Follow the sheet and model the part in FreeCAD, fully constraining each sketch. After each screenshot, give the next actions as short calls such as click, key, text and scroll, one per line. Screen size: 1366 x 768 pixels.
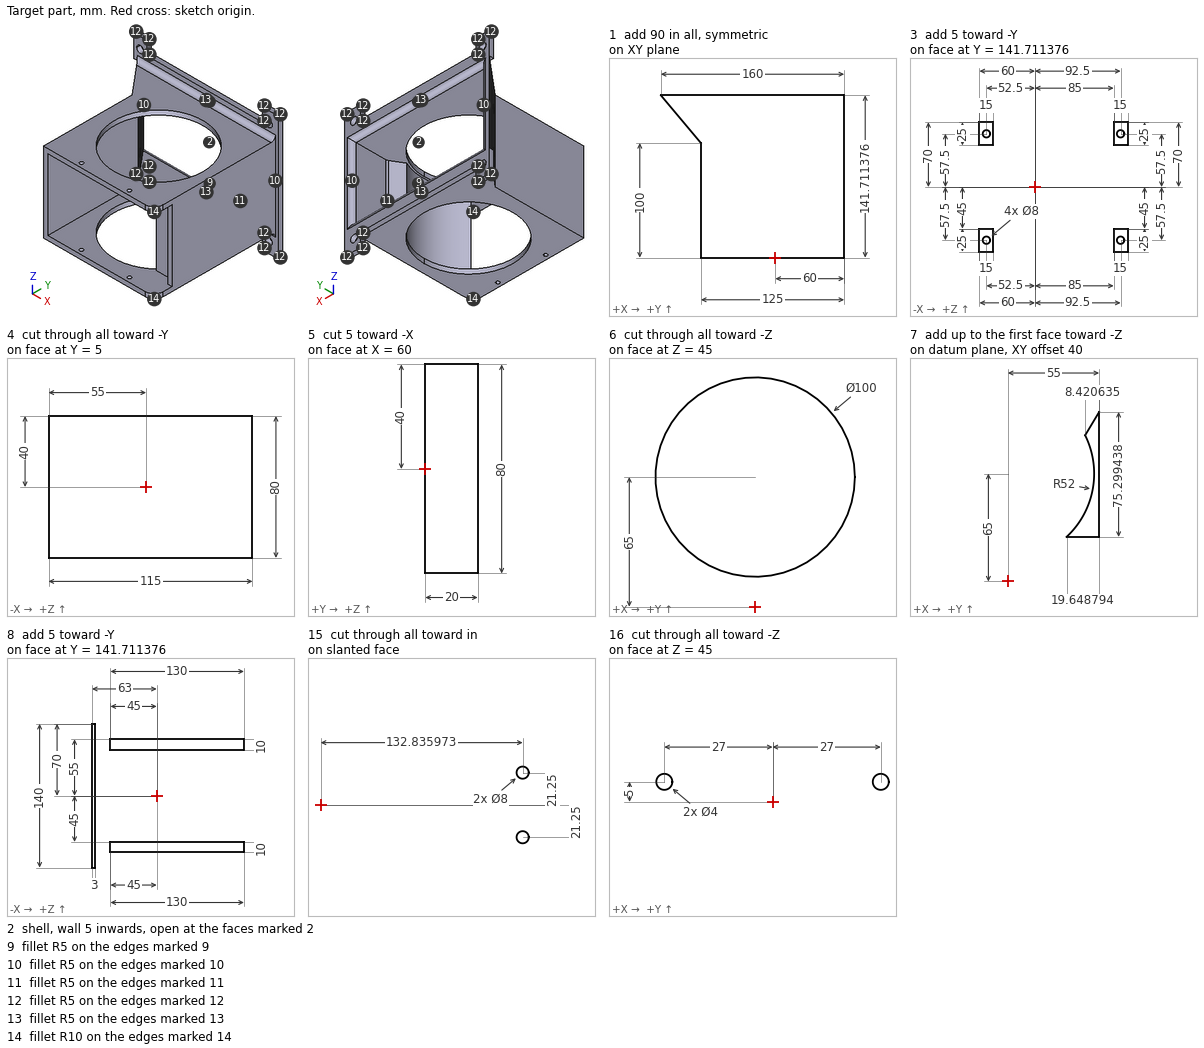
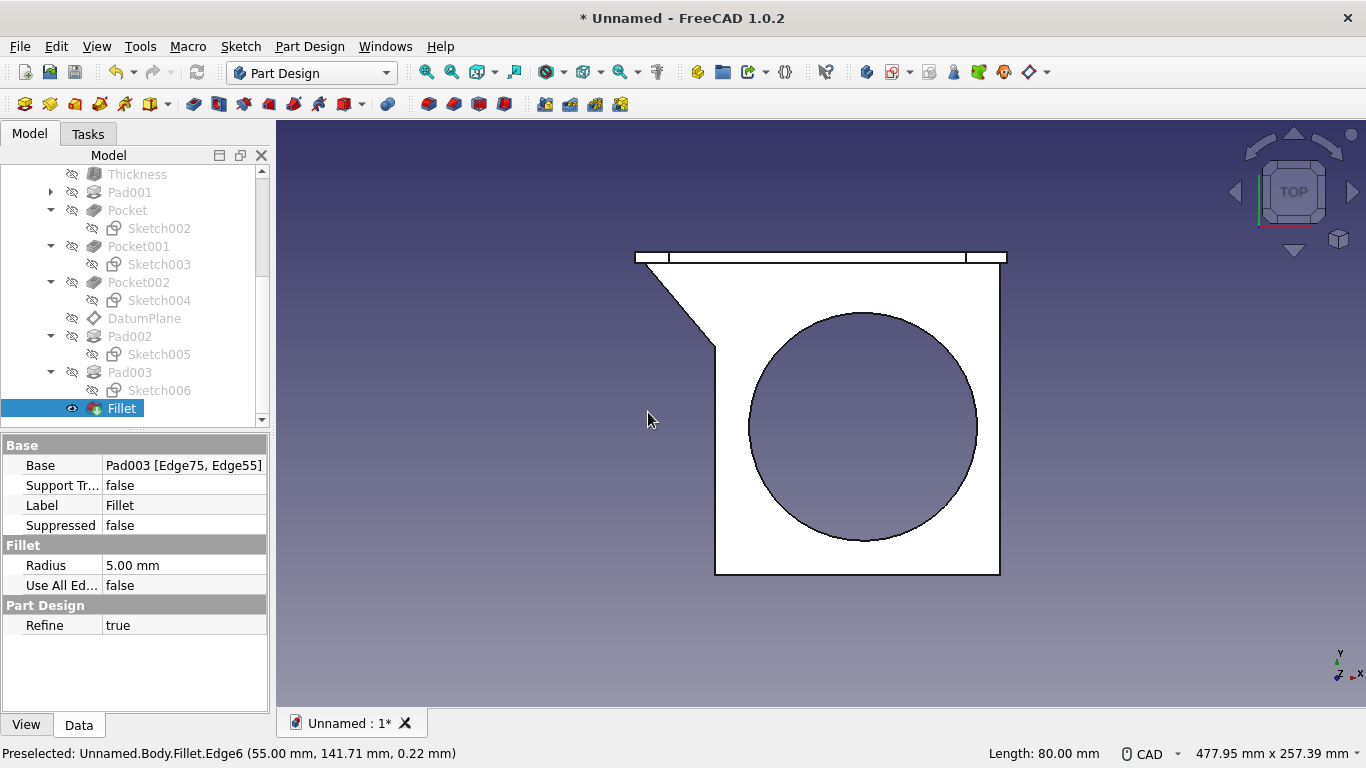
key(1)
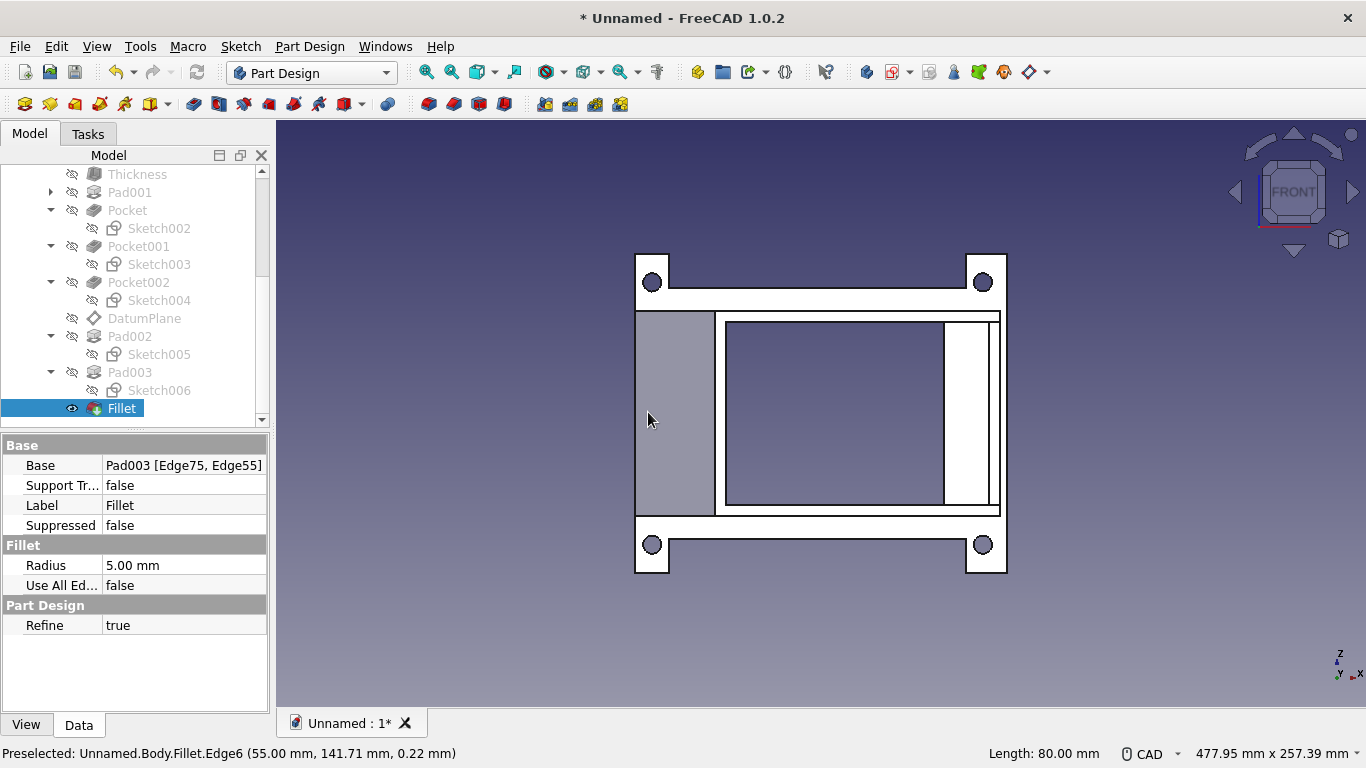
key(3)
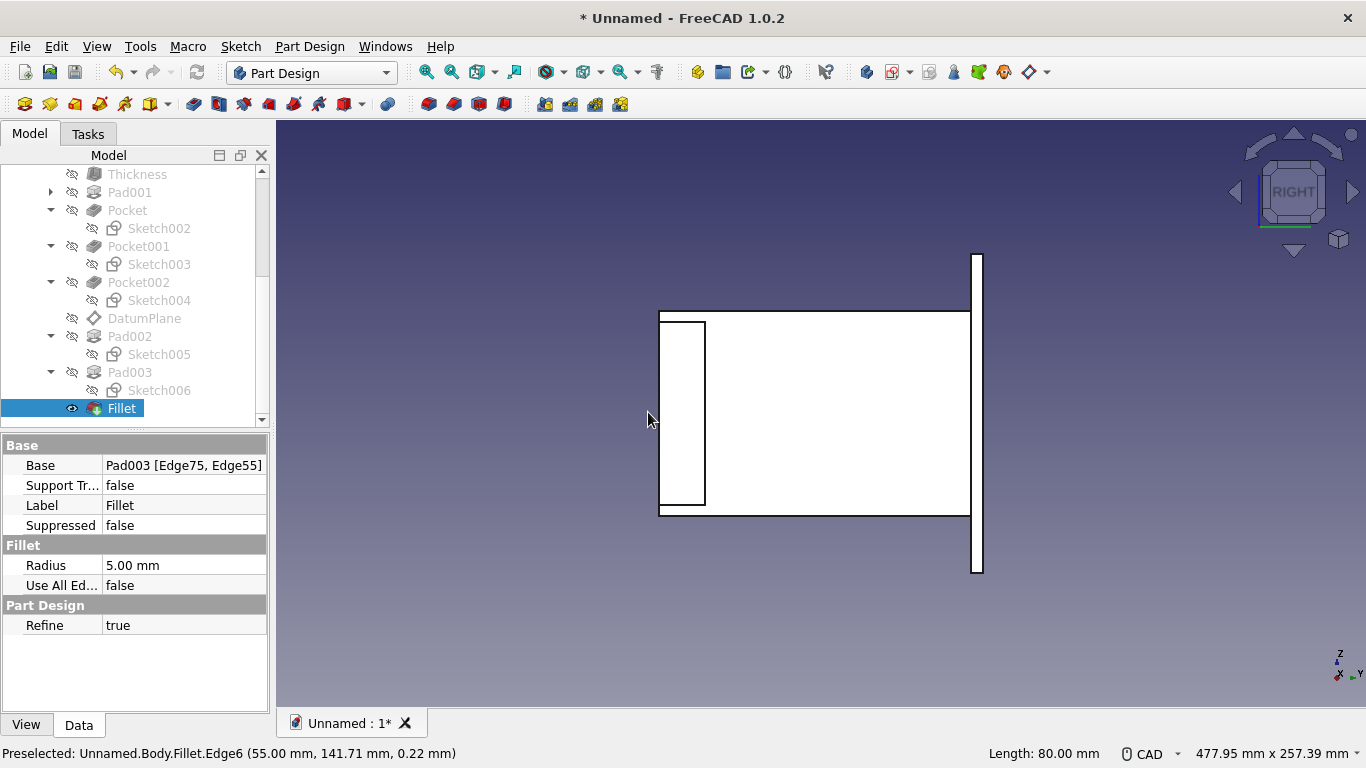
key(5)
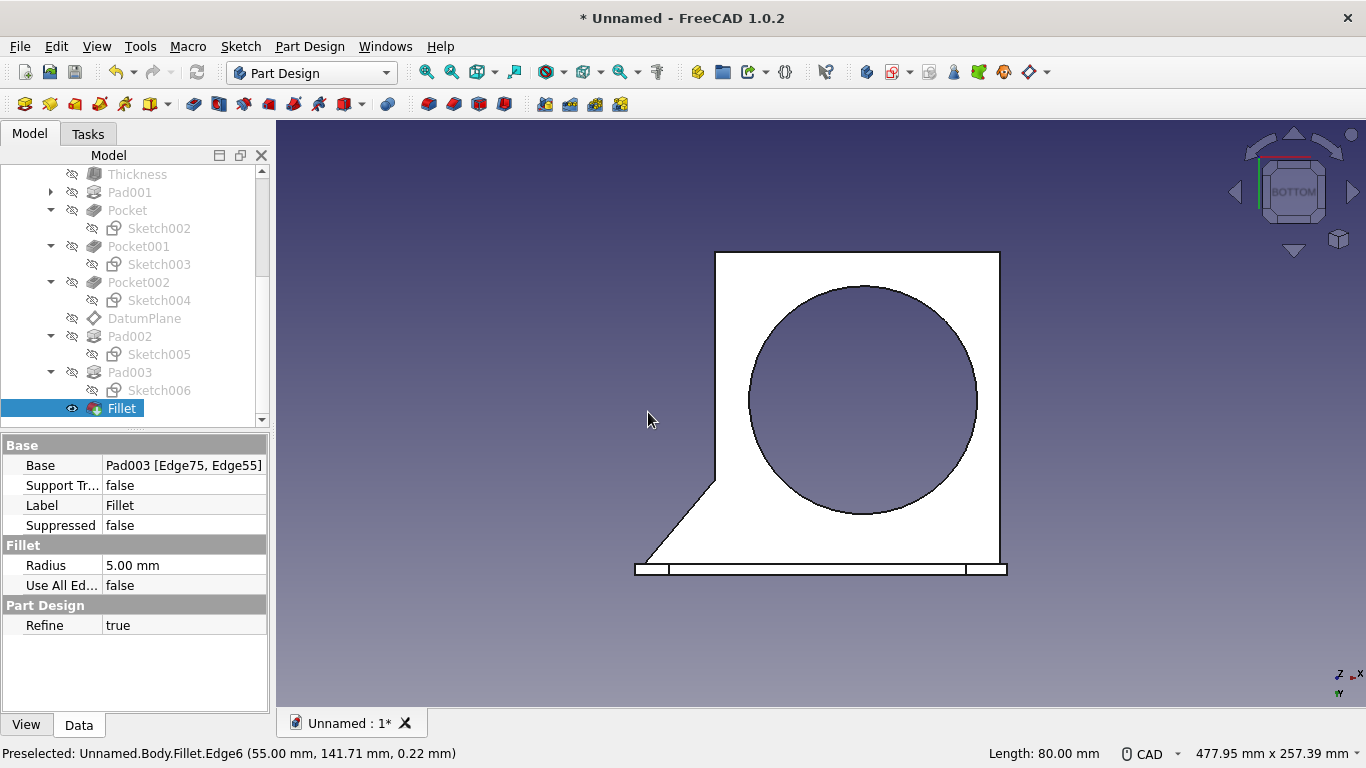
key(4)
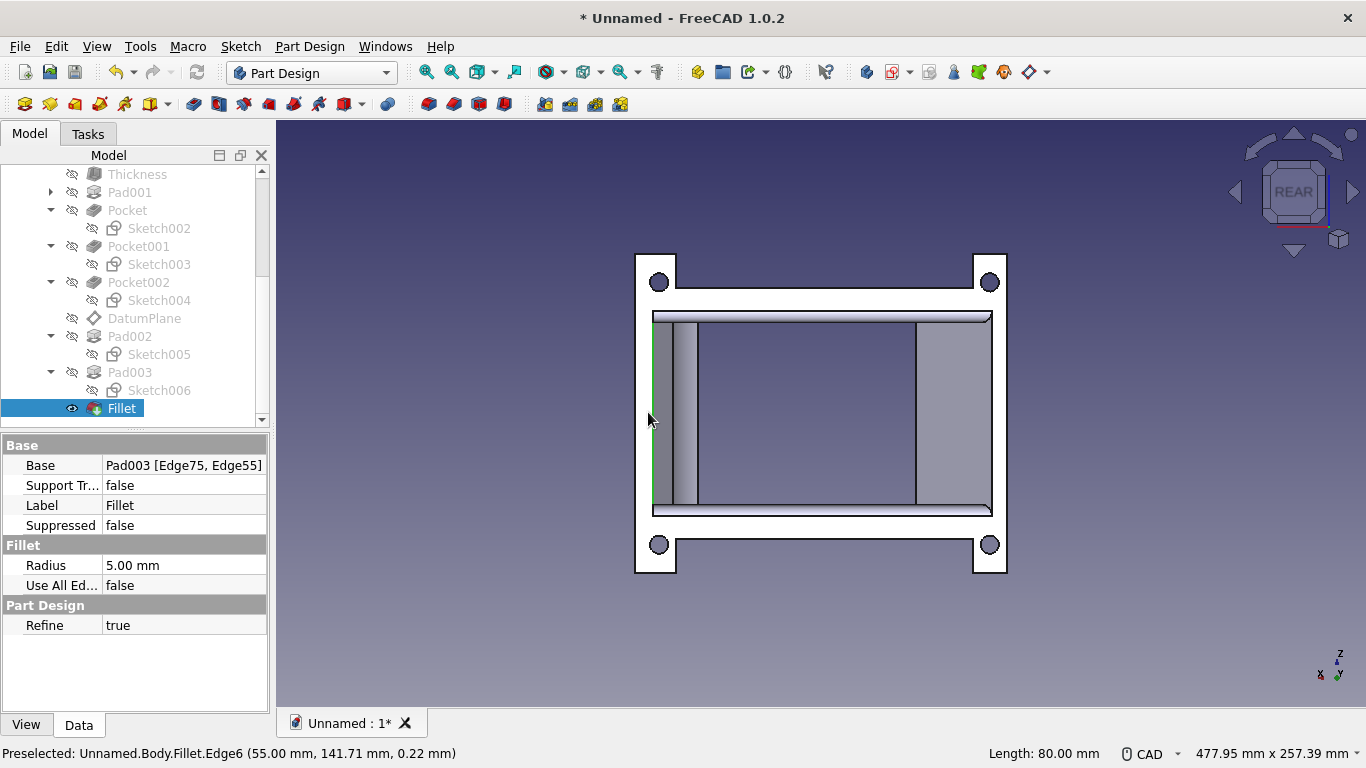
click(992, 412, ctrl)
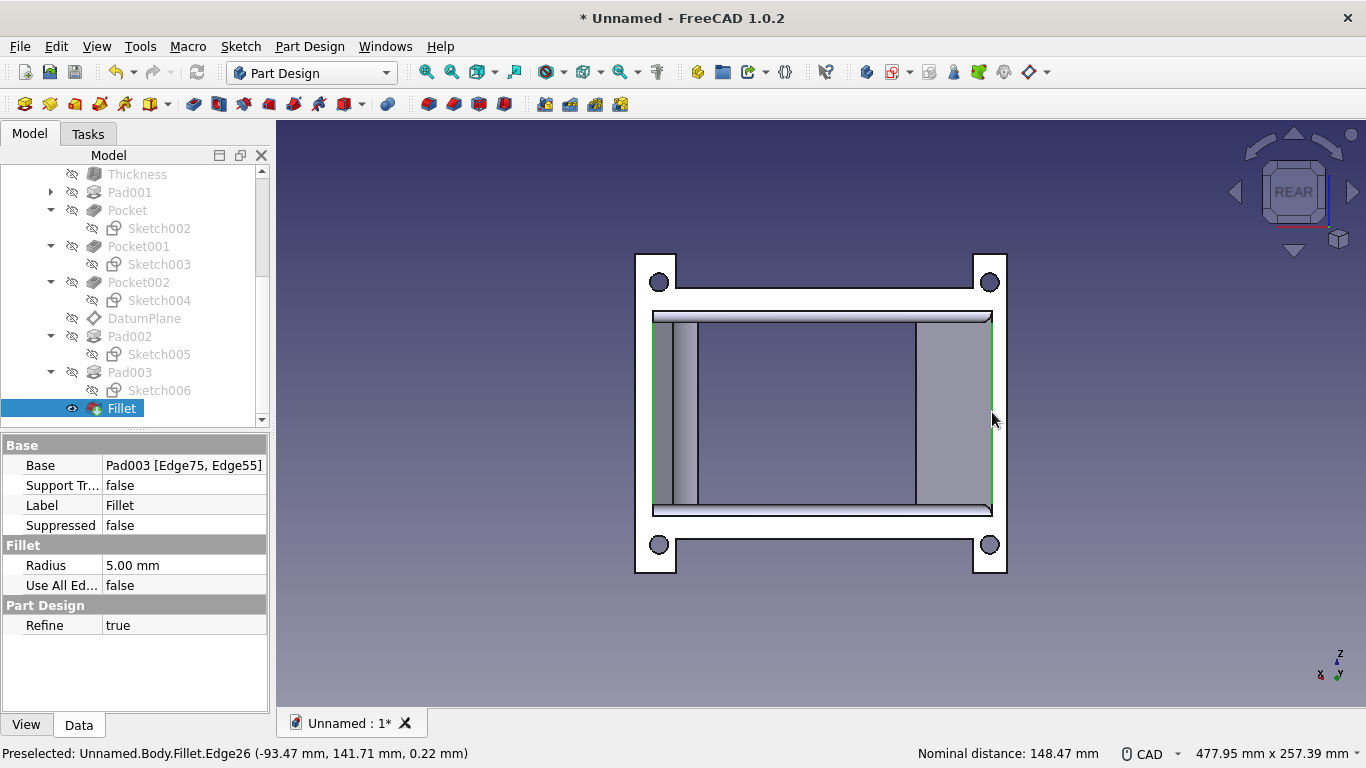
click(429, 104)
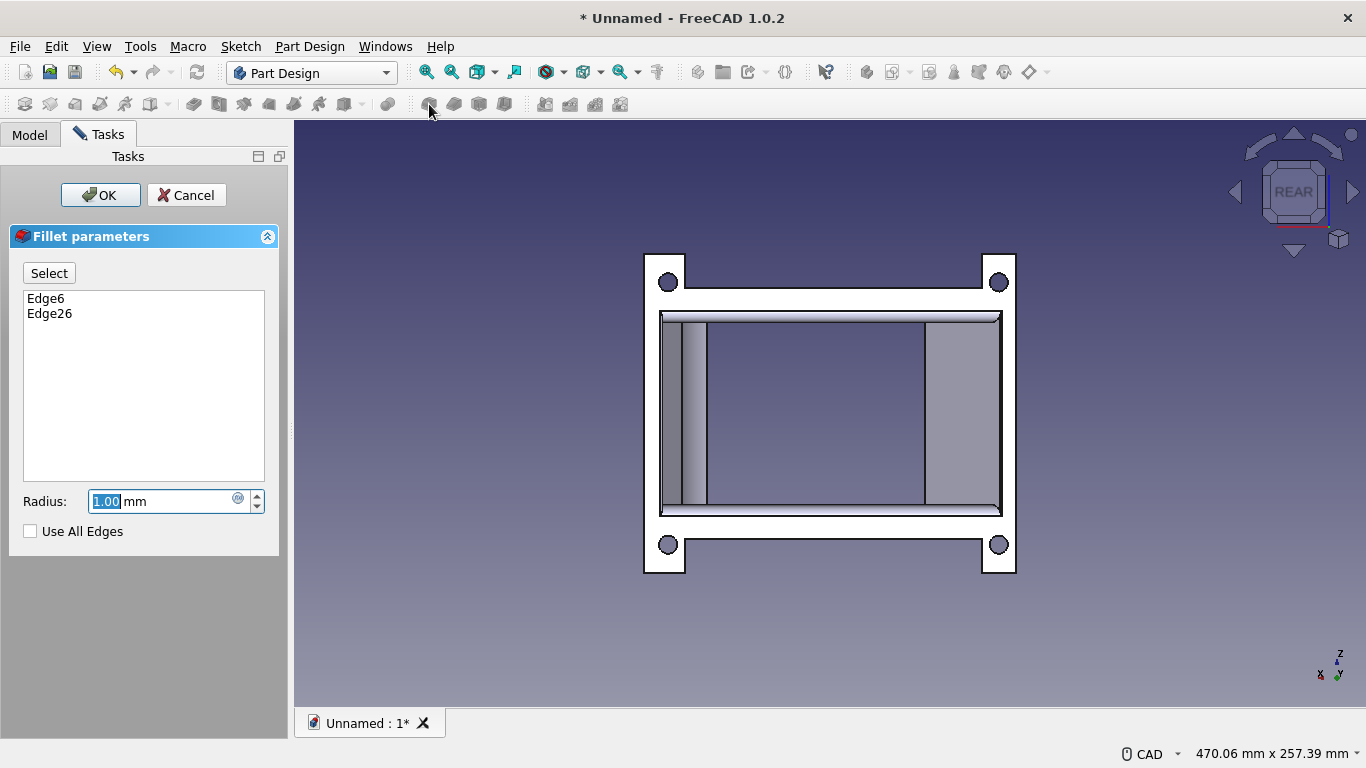
text(5)
key(Tab)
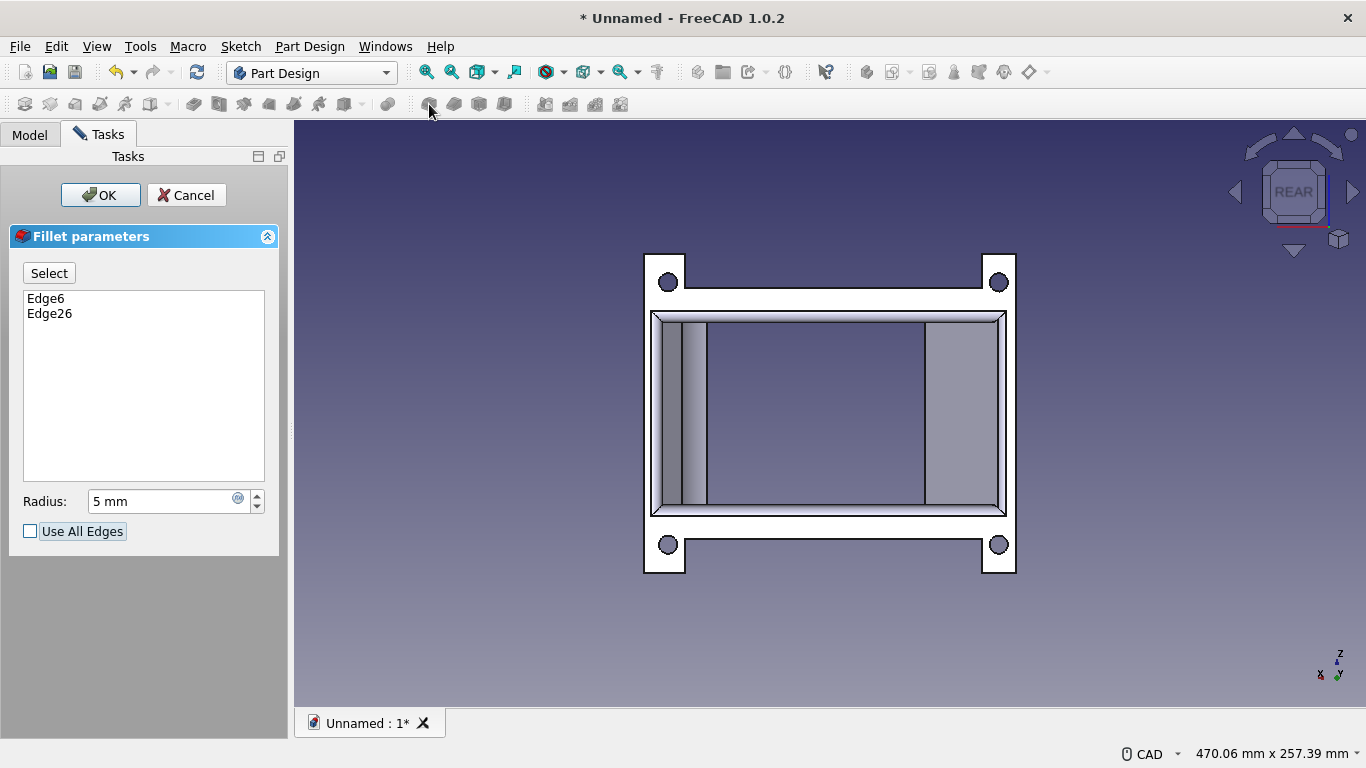
click(101, 195)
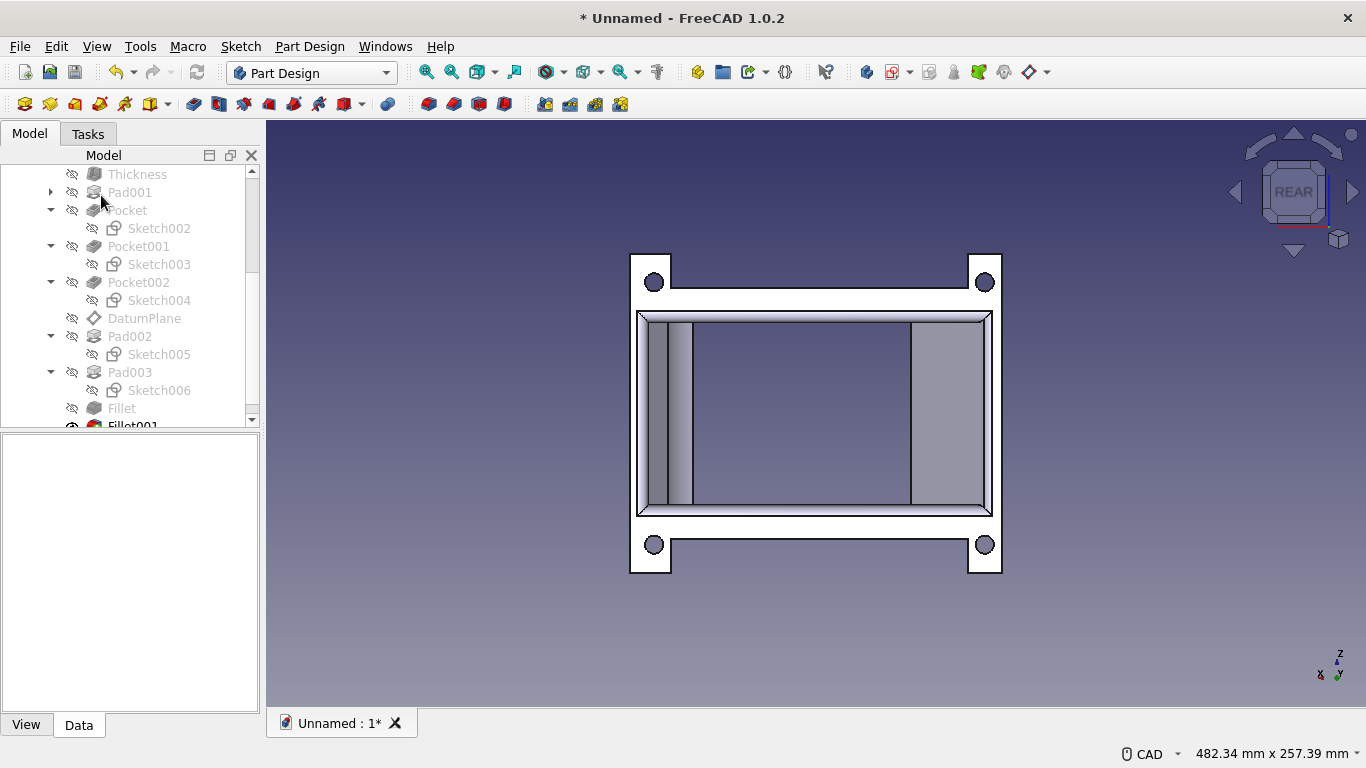
key(0)